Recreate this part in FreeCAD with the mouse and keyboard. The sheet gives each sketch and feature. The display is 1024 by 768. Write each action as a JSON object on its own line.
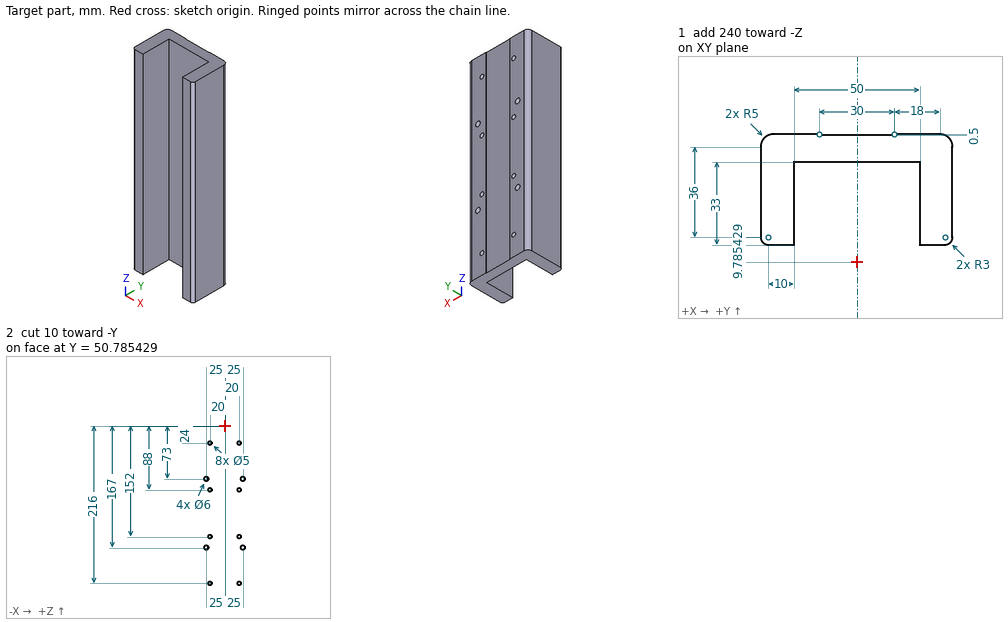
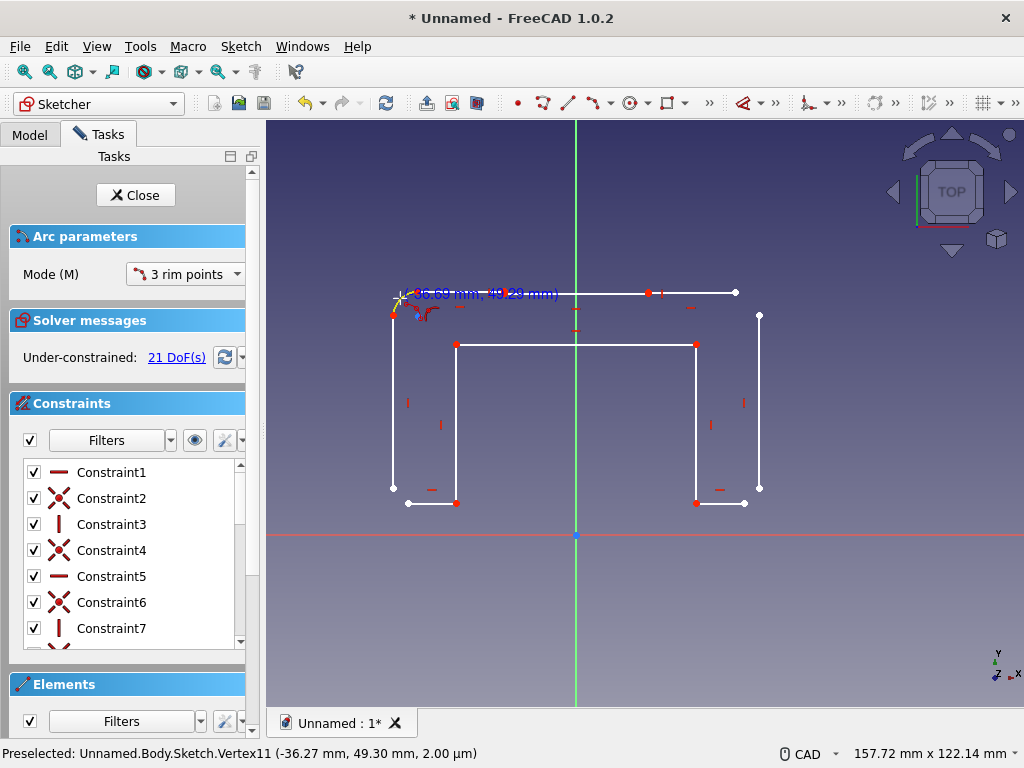
{"action": "left_click", "coordinate": [393, 489]}
{"action": "left_click", "coordinate": [408, 504]}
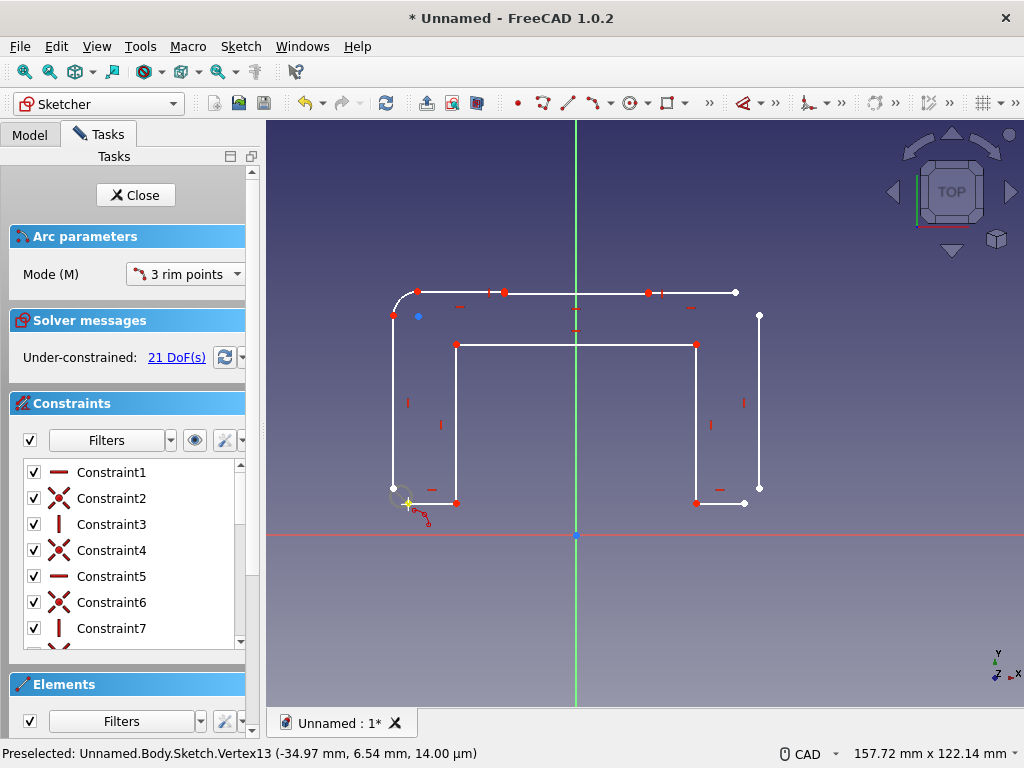
{"action": "scroll", "coordinate": [398, 499], "scroll_direction": "up", "scroll_amount": 7}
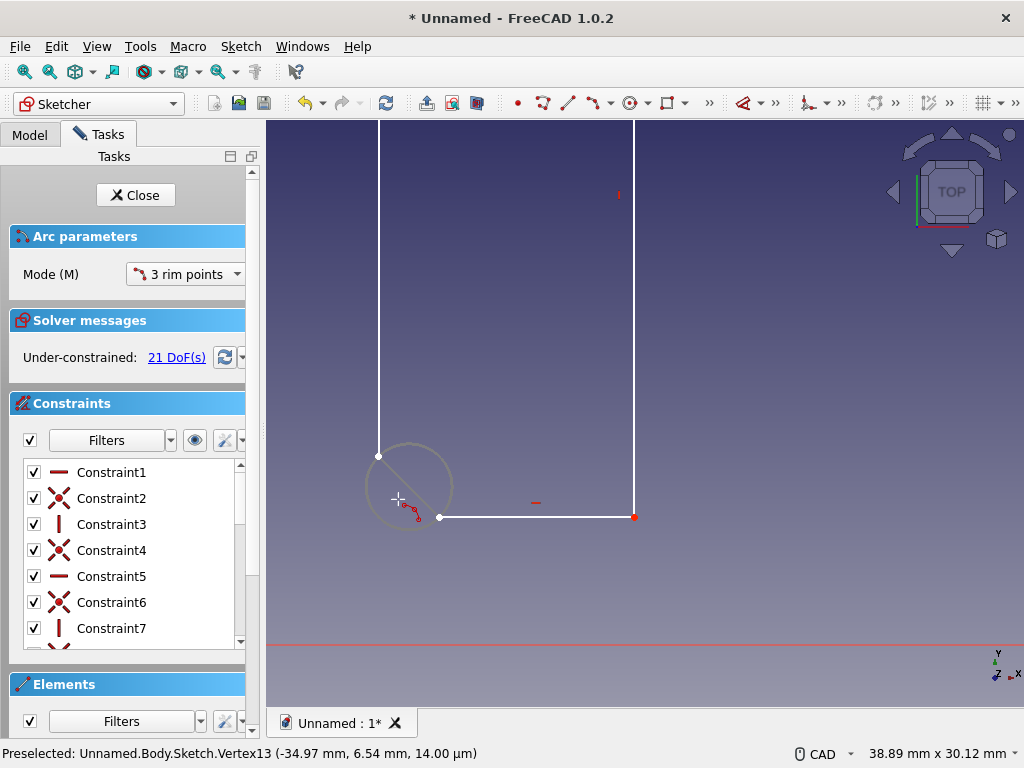
{"action": "left_click", "coordinate": [398, 495]}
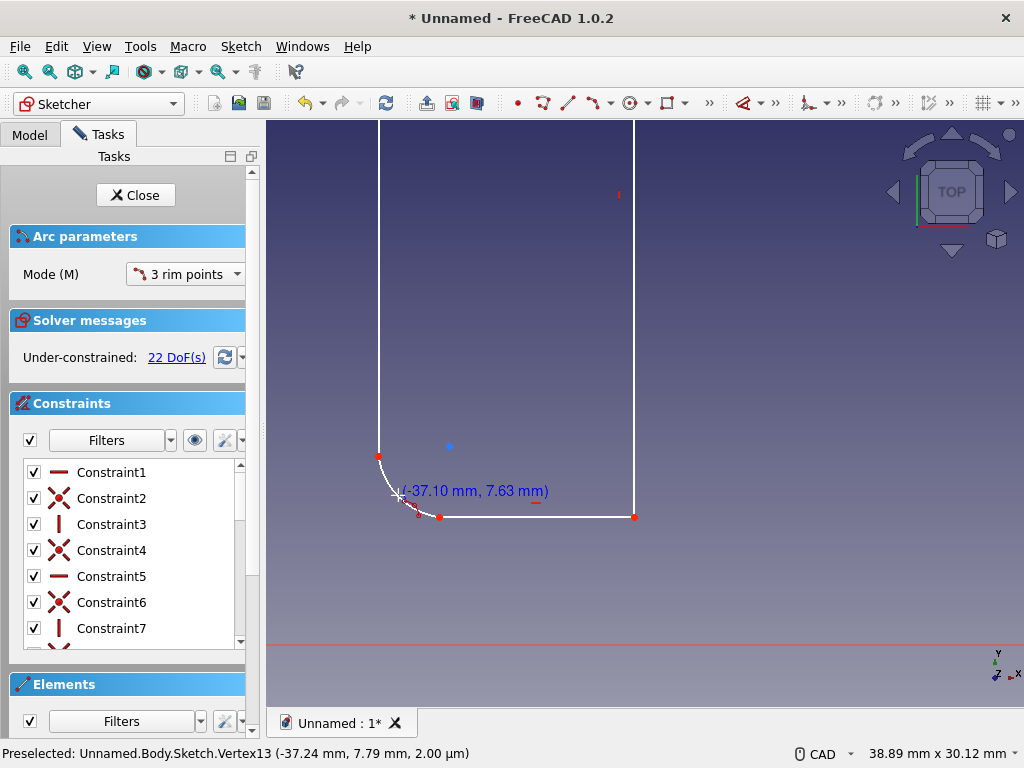
{"action": "scroll", "coordinate": [398, 500], "scroll_direction": "down", "scroll_amount": 7}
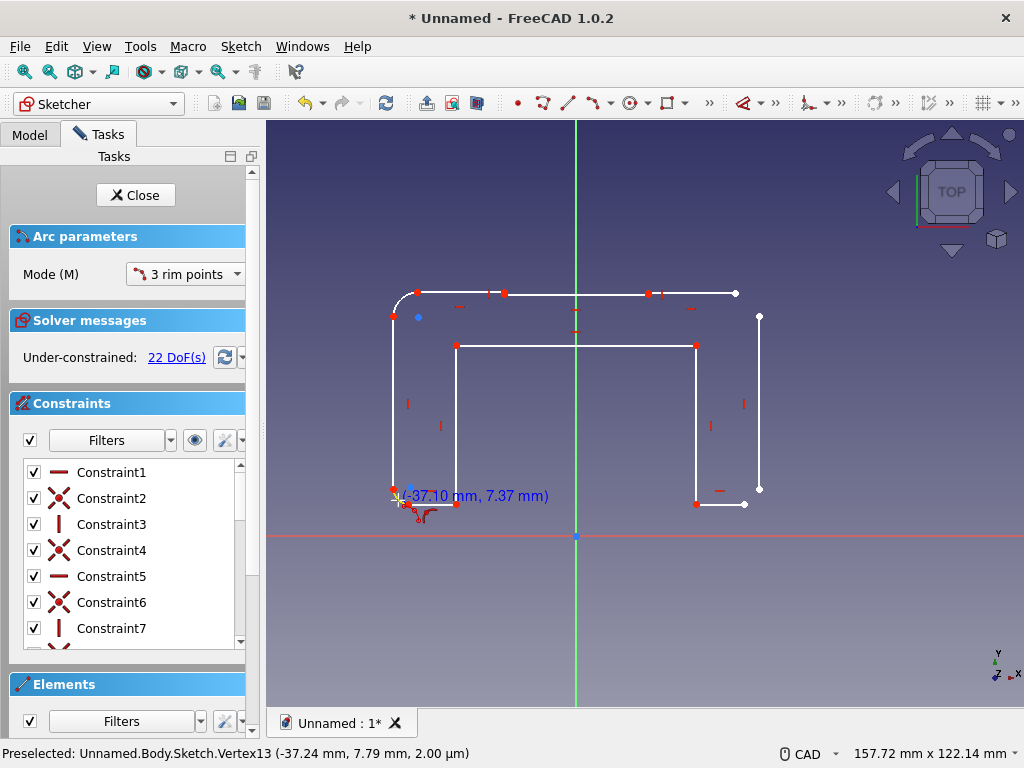
{"action": "left_click", "coordinate": [744, 505]}
{"action": "left_click", "coordinate": [759, 490]}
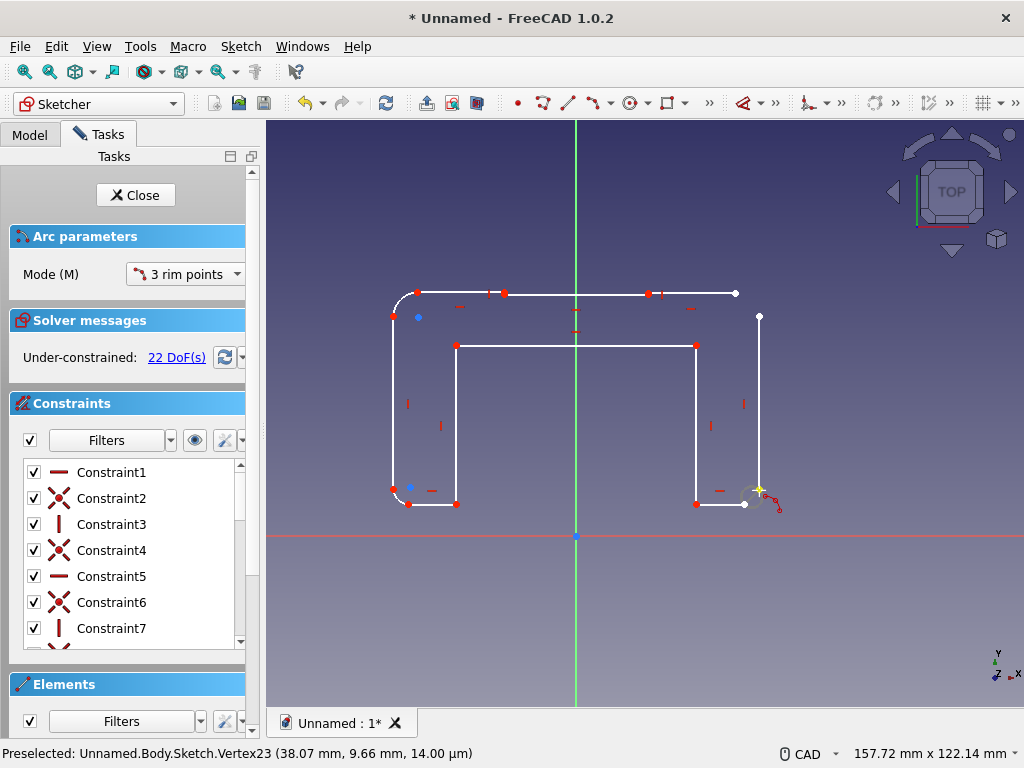
{"action": "scroll", "coordinate": [755, 499], "scroll_direction": "up", "scroll_amount": 7}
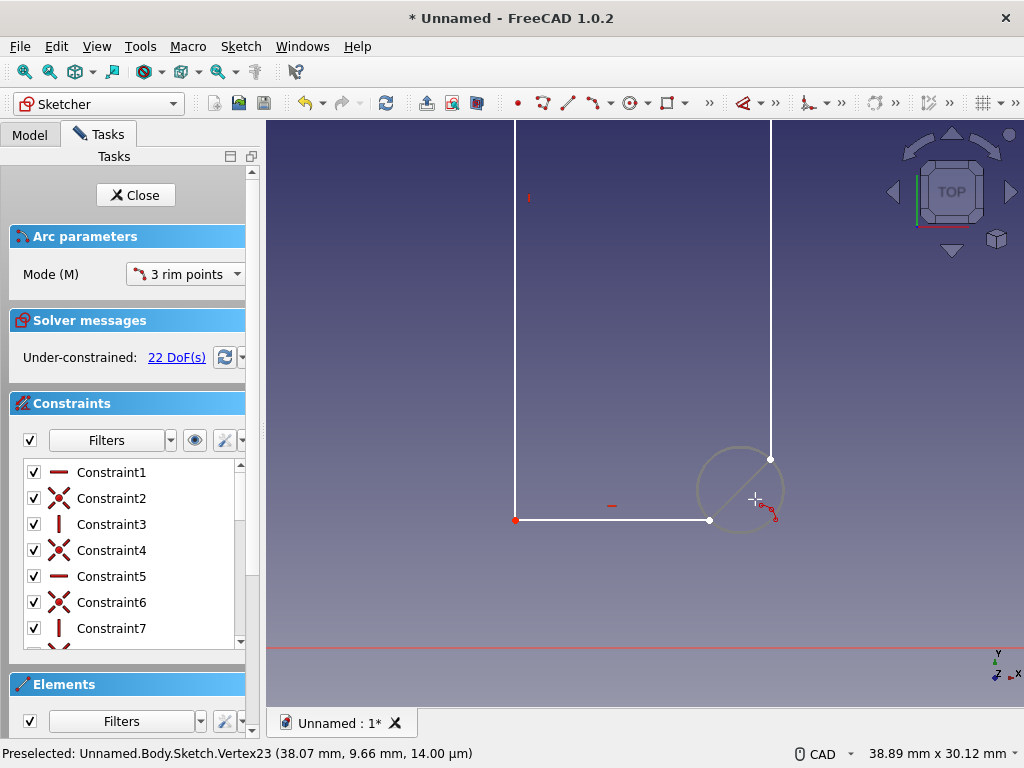
{"action": "left_click", "coordinate": [752, 498]}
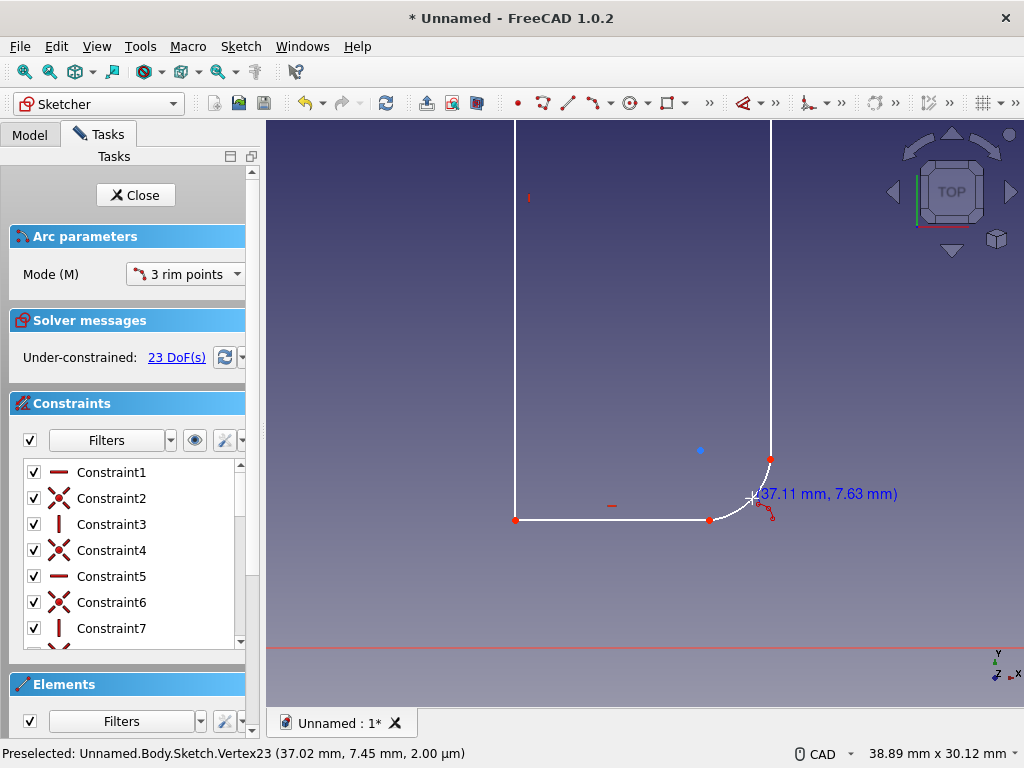
{"action": "scroll", "coordinate": [756, 499], "scroll_direction": "down", "scroll_amount": 7}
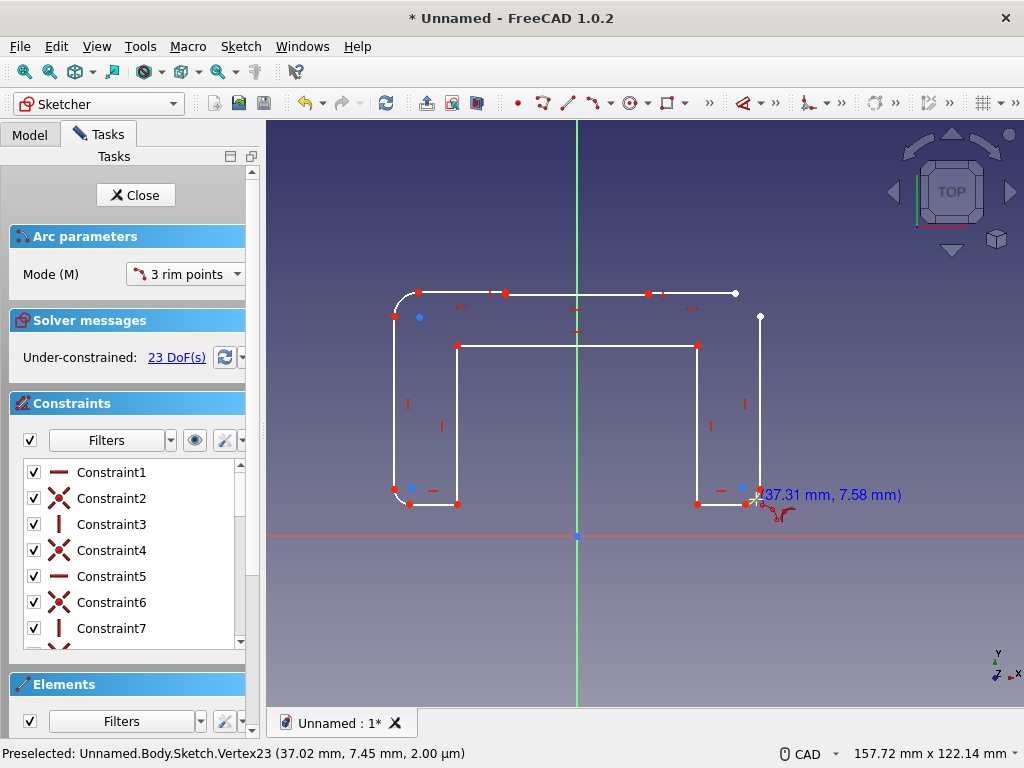
{"action": "left_click", "coordinate": [760, 317]}
{"action": "left_click", "coordinate": [736, 293]}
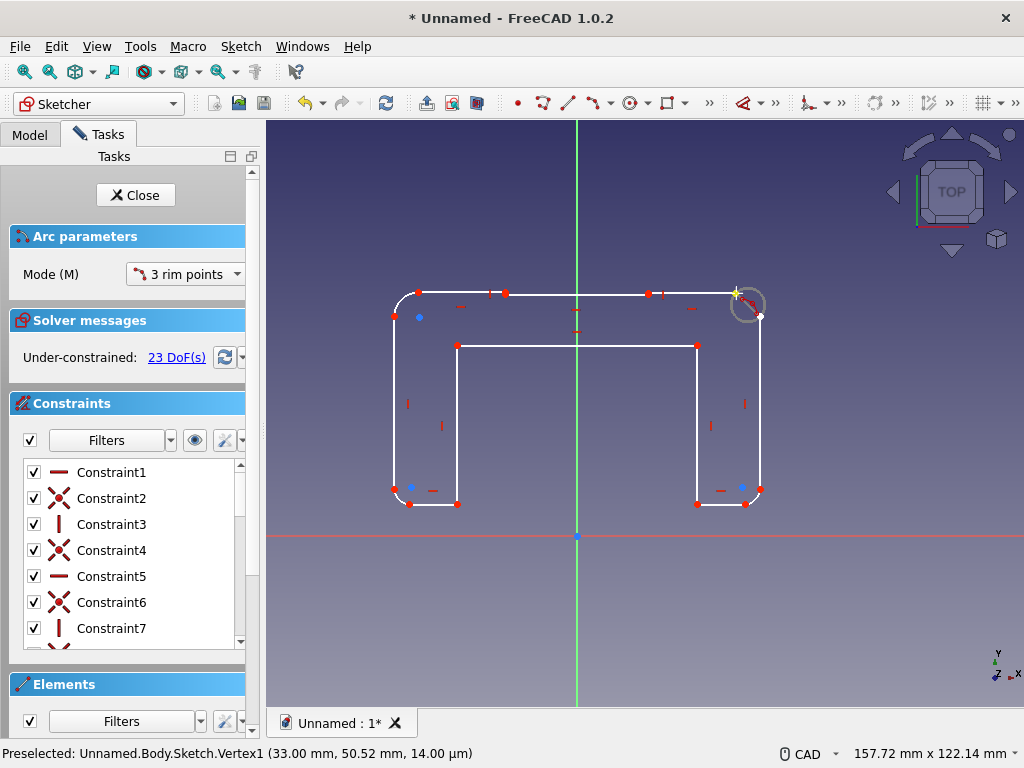
{"action": "scroll", "coordinate": [753, 299], "scroll_direction": "up", "scroll_amount": 5}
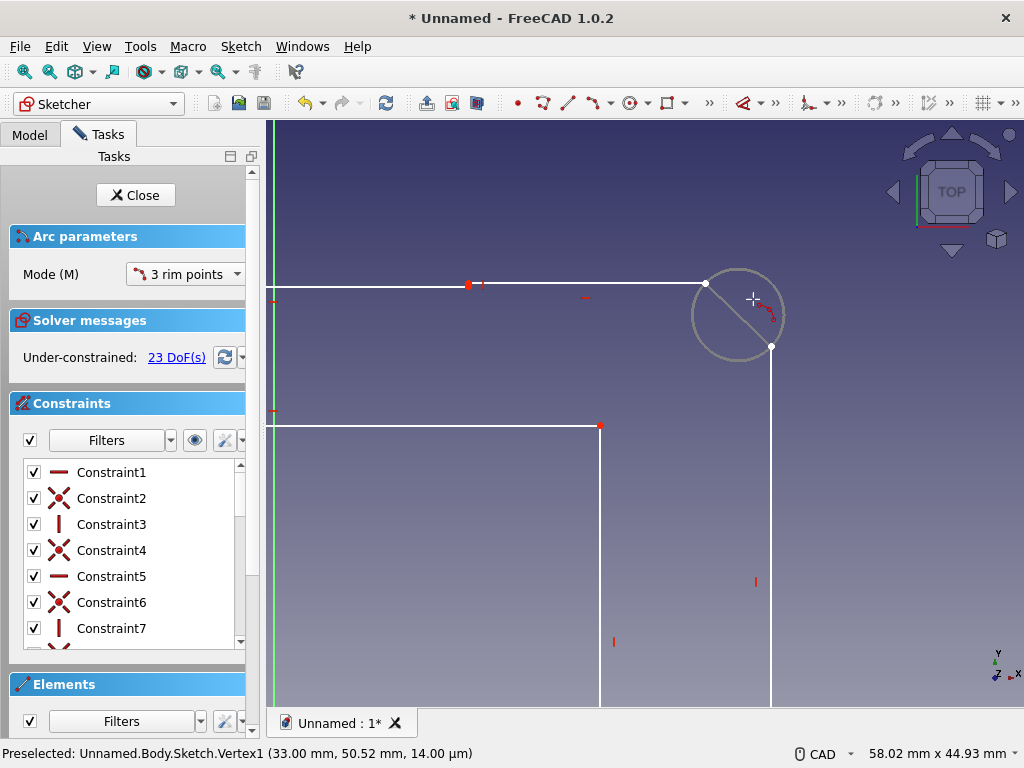
{"action": "left_click", "coordinate": [751, 299]}
{"action": "key", "text": "Escape"}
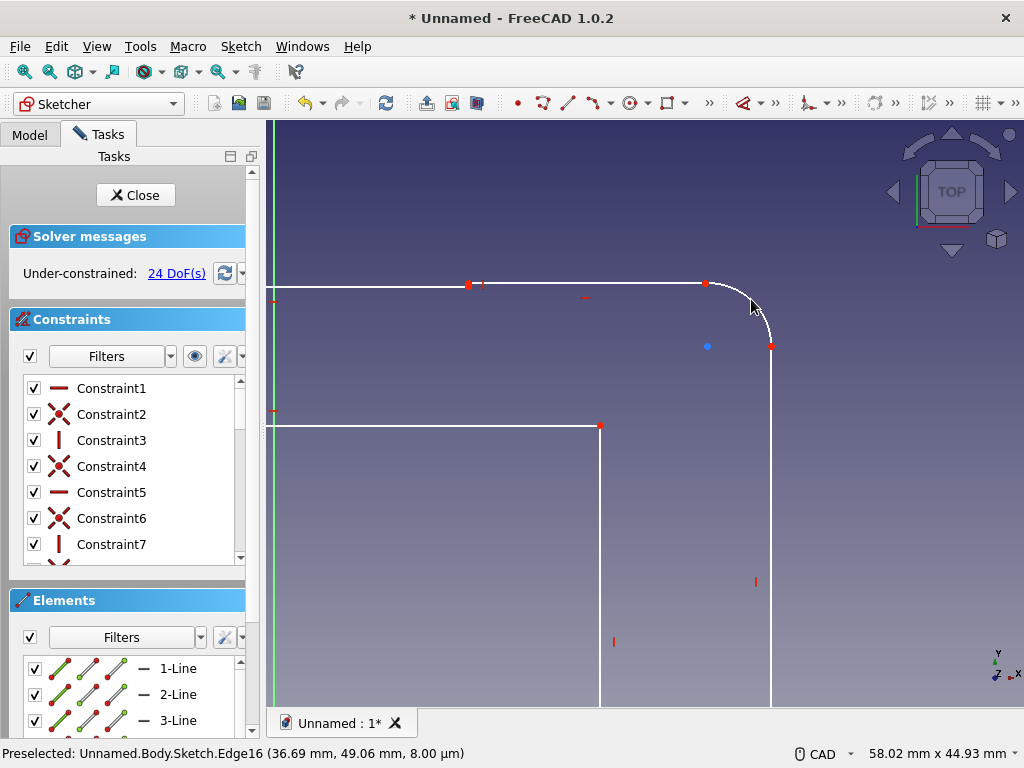
{"action": "left_click", "coordinate": [634, 283]}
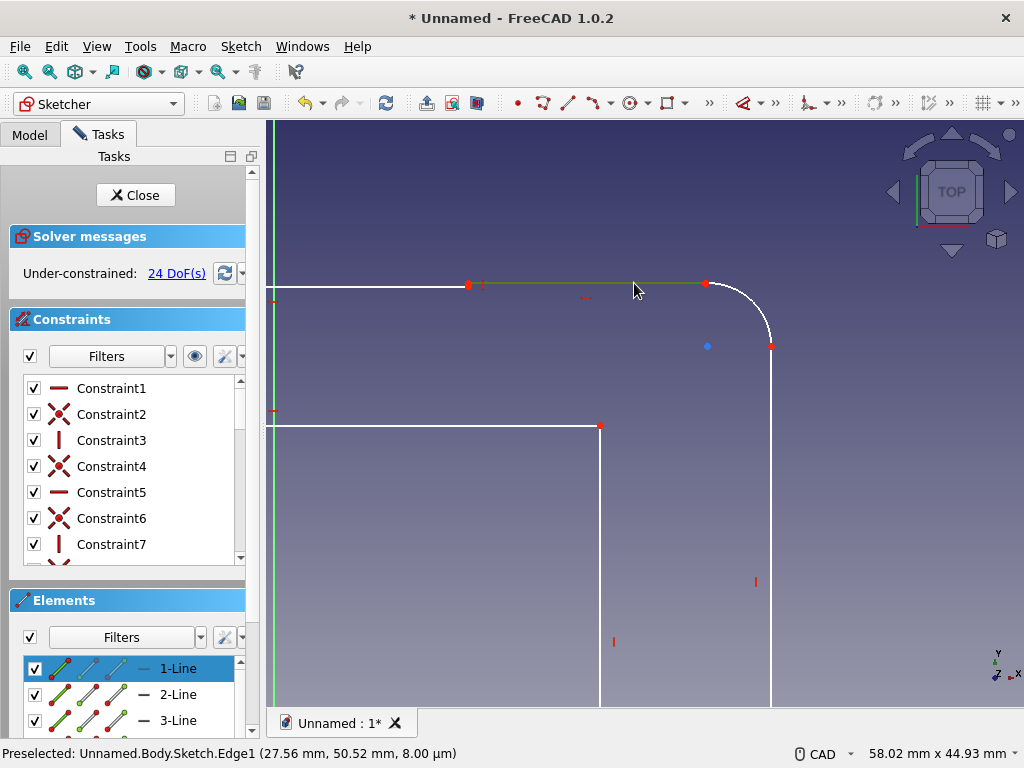
{"action": "left_click", "coordinate": [764, 317]}